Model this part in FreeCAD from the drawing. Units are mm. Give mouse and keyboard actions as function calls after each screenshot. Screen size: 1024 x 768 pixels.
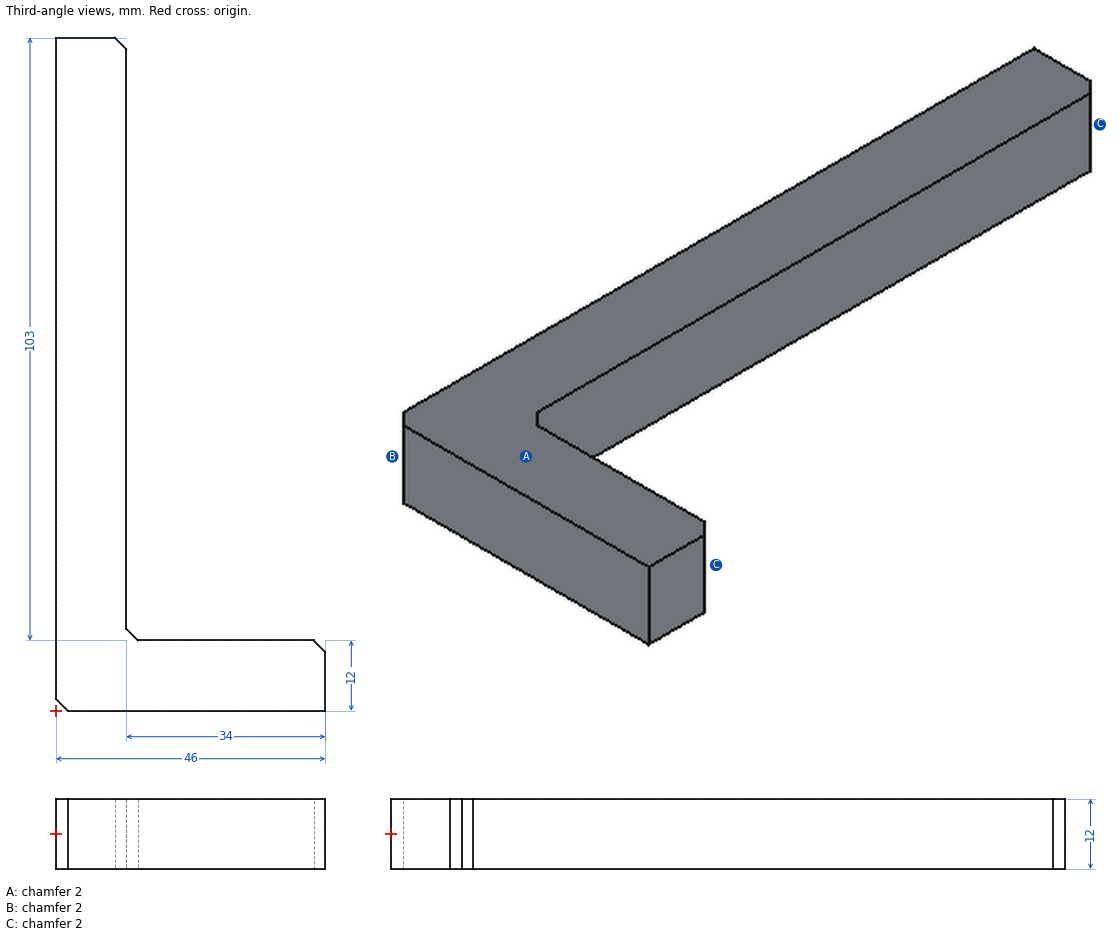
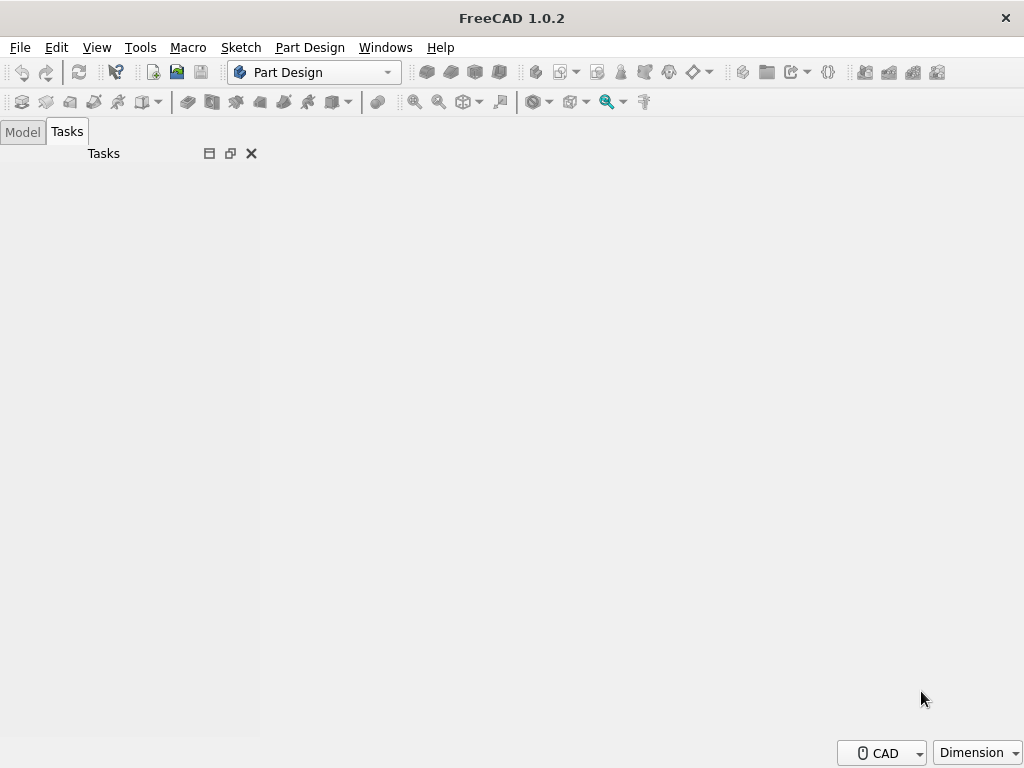
click(154, 72)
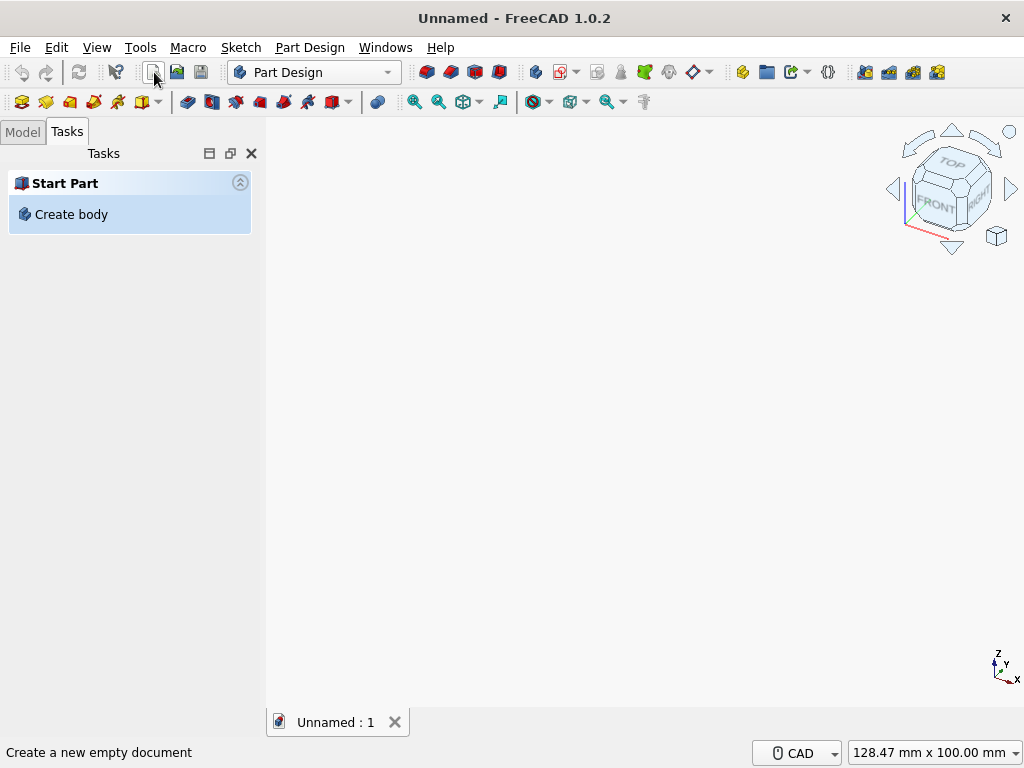
click(560, 72)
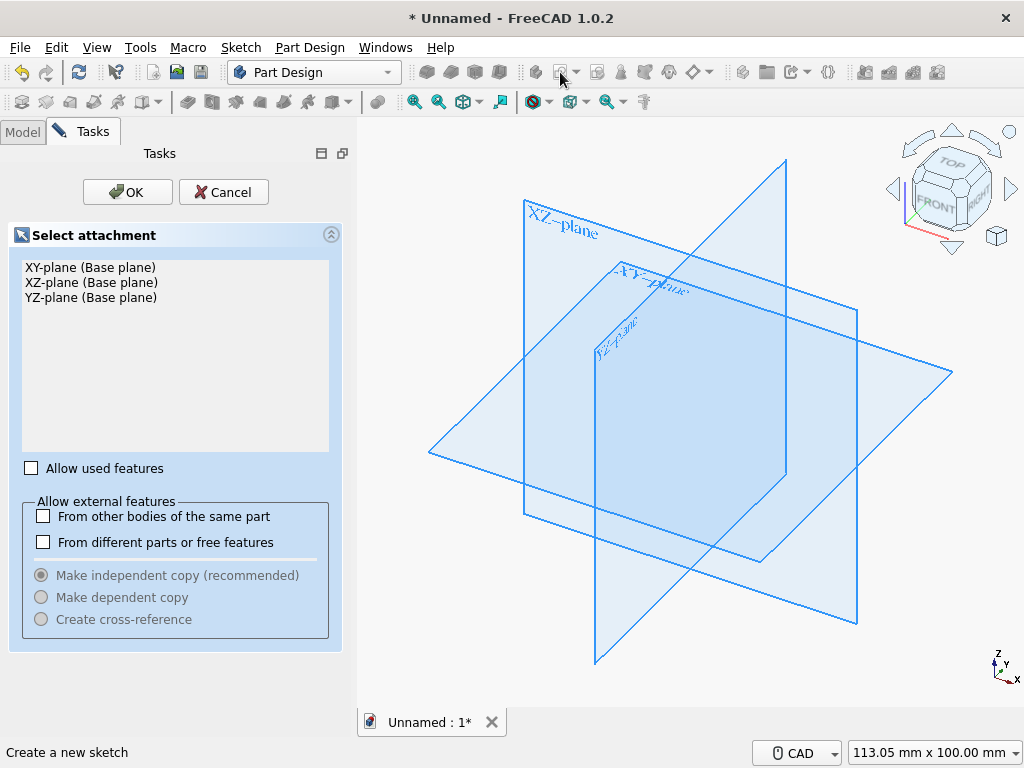
click(82, 268)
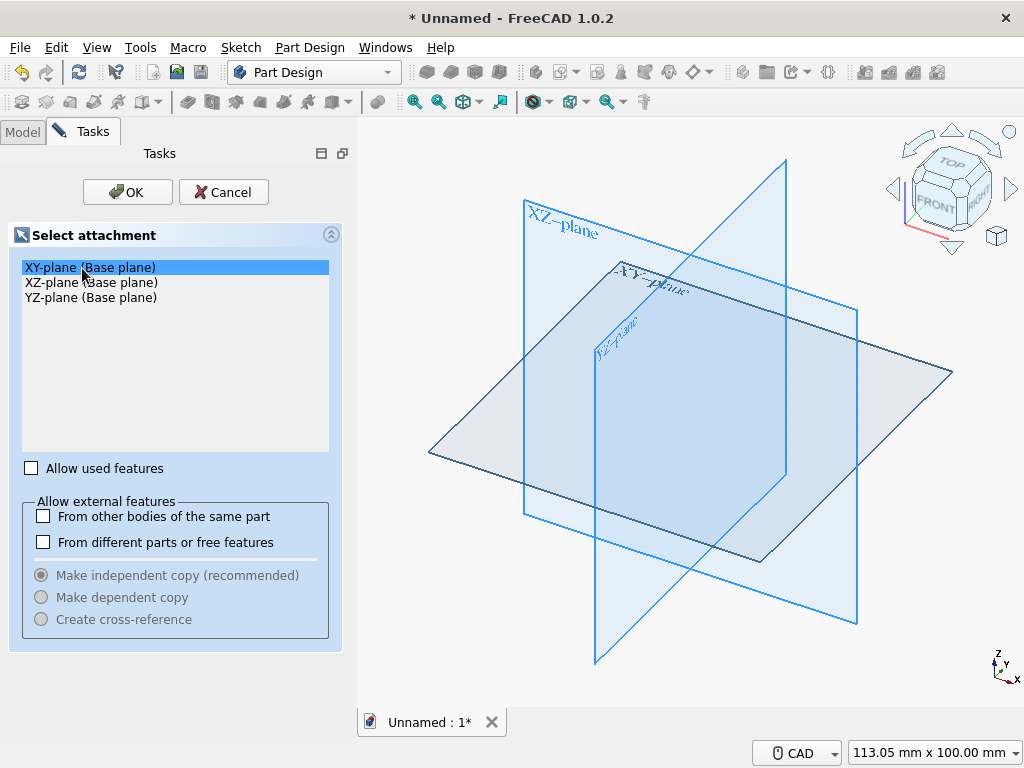
click(128, 192)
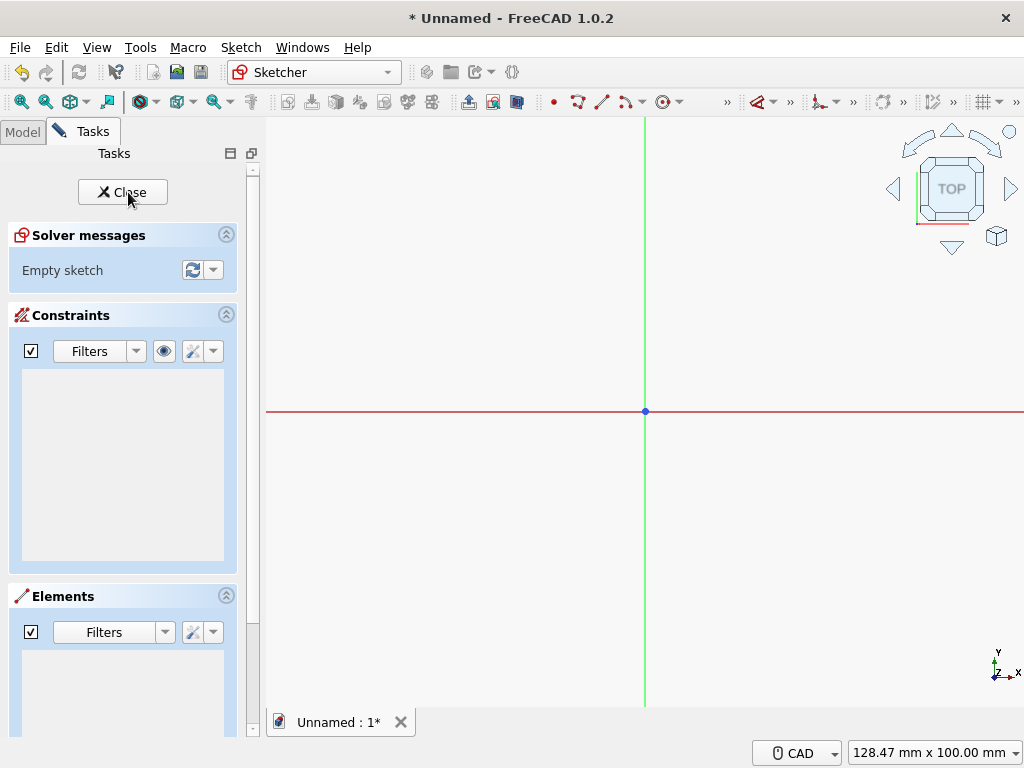
scroll(410, 679, down, 4)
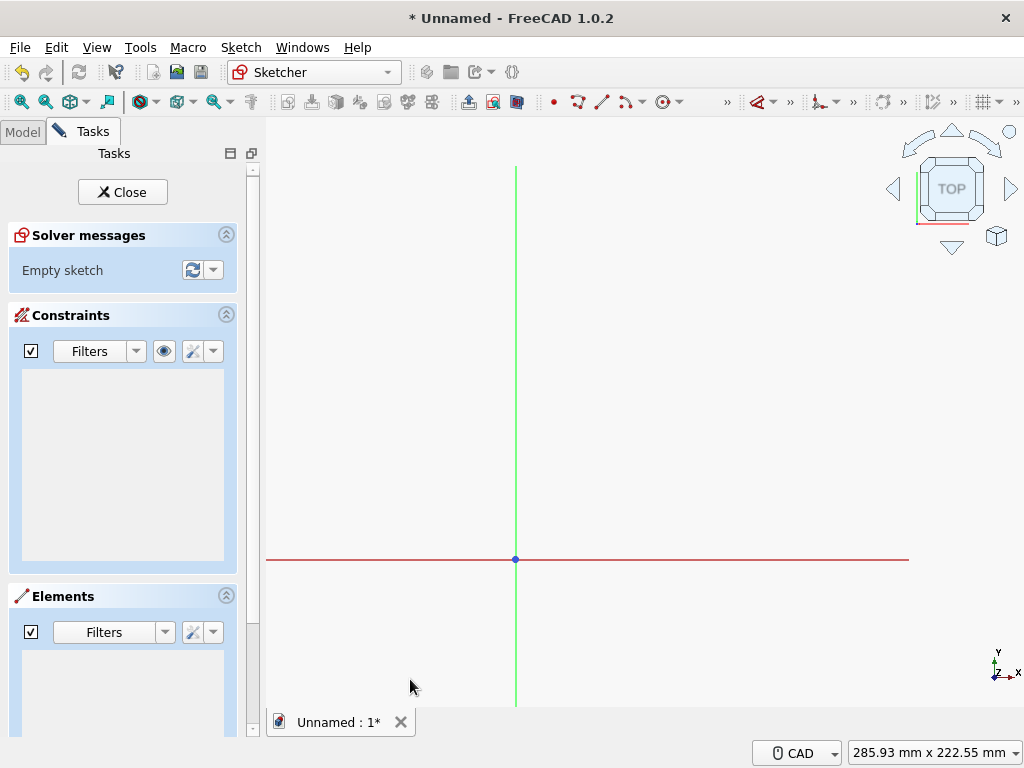
click(578, 102)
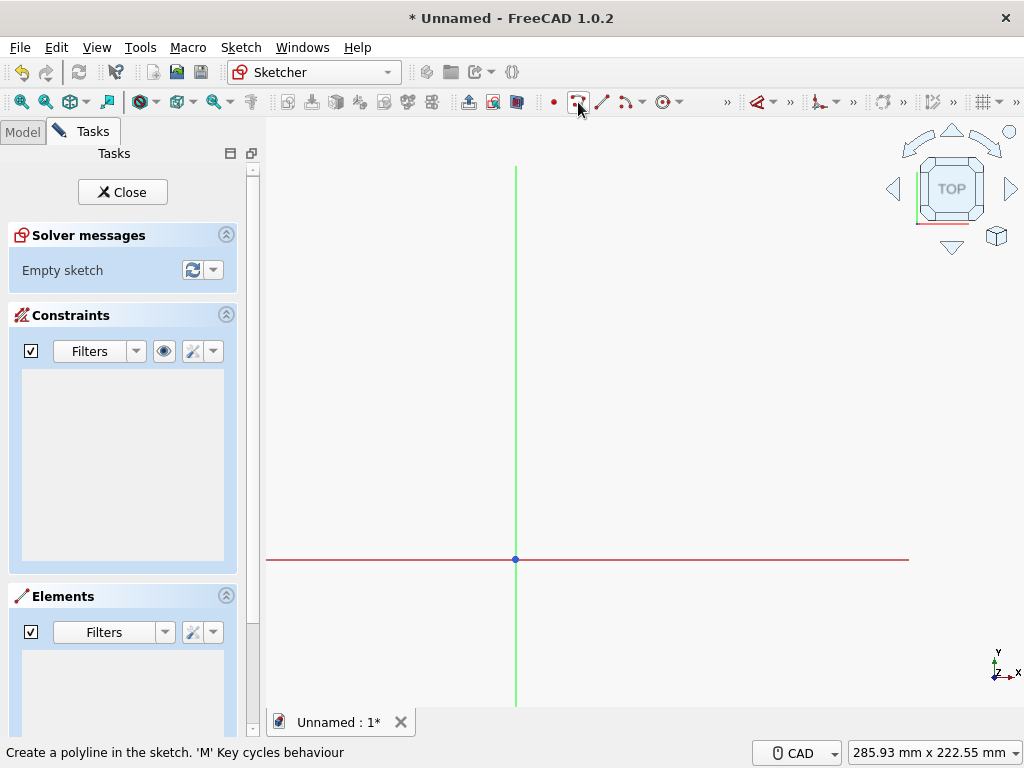
click(516, 560)
click(638, 551)
click(638, 528)
click(548, 528)
click(548, 255)
click(525, 255)
click(516, 560)
key(Escape)
key(Escape)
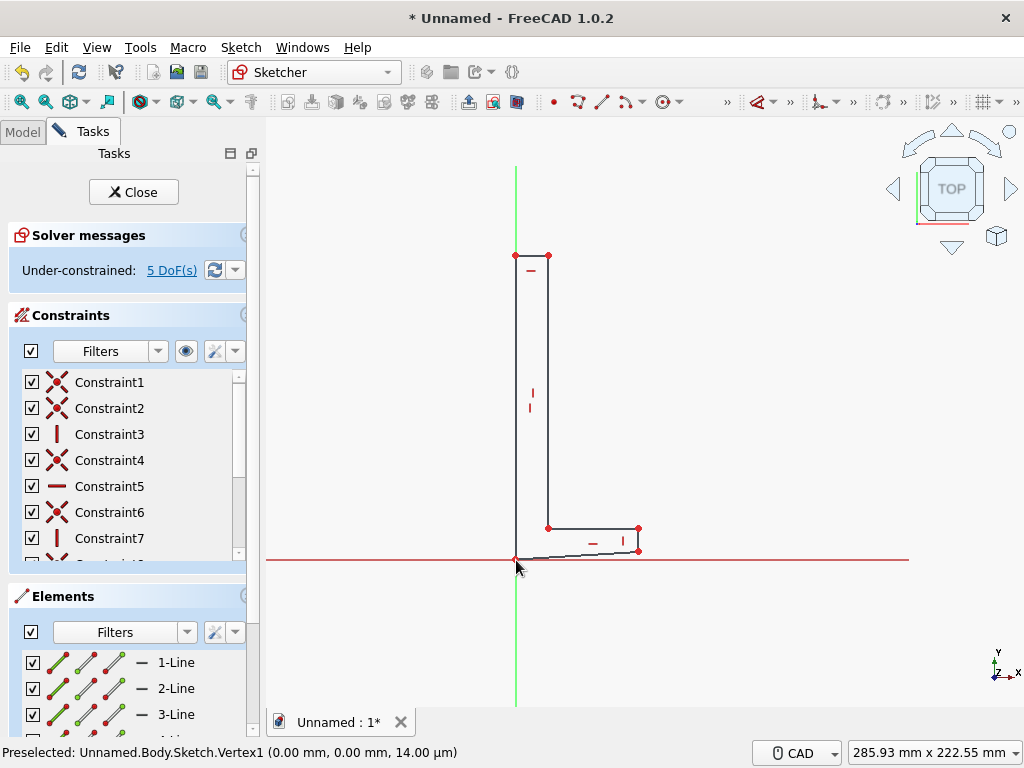
click(552, 557)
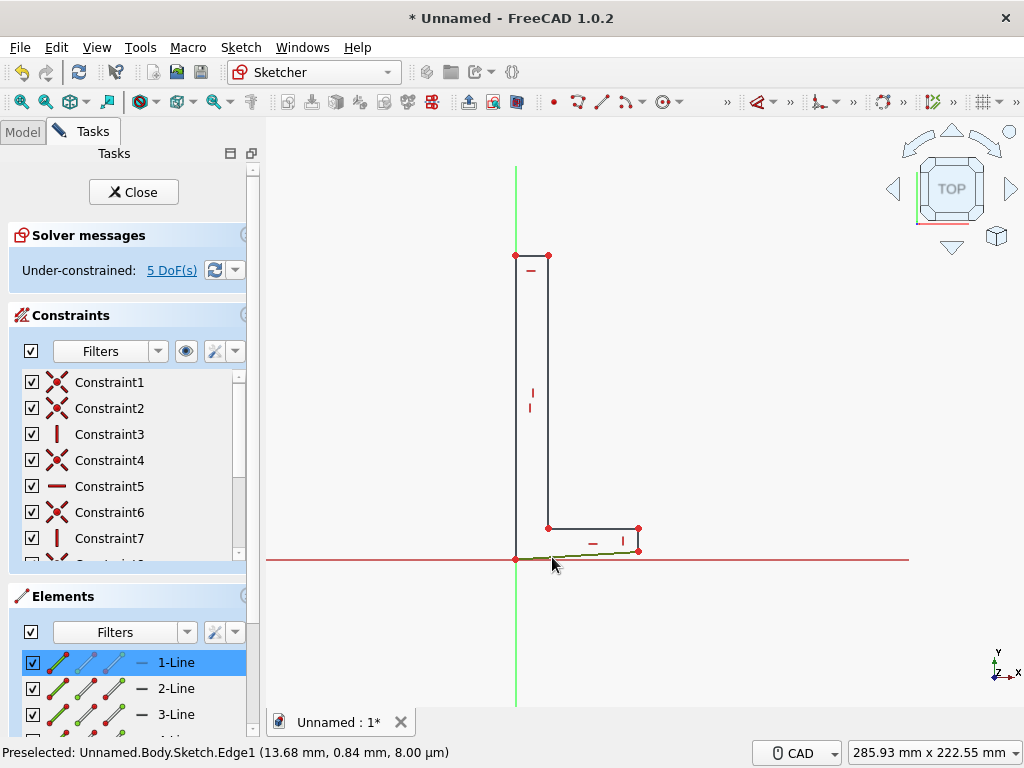
key(h)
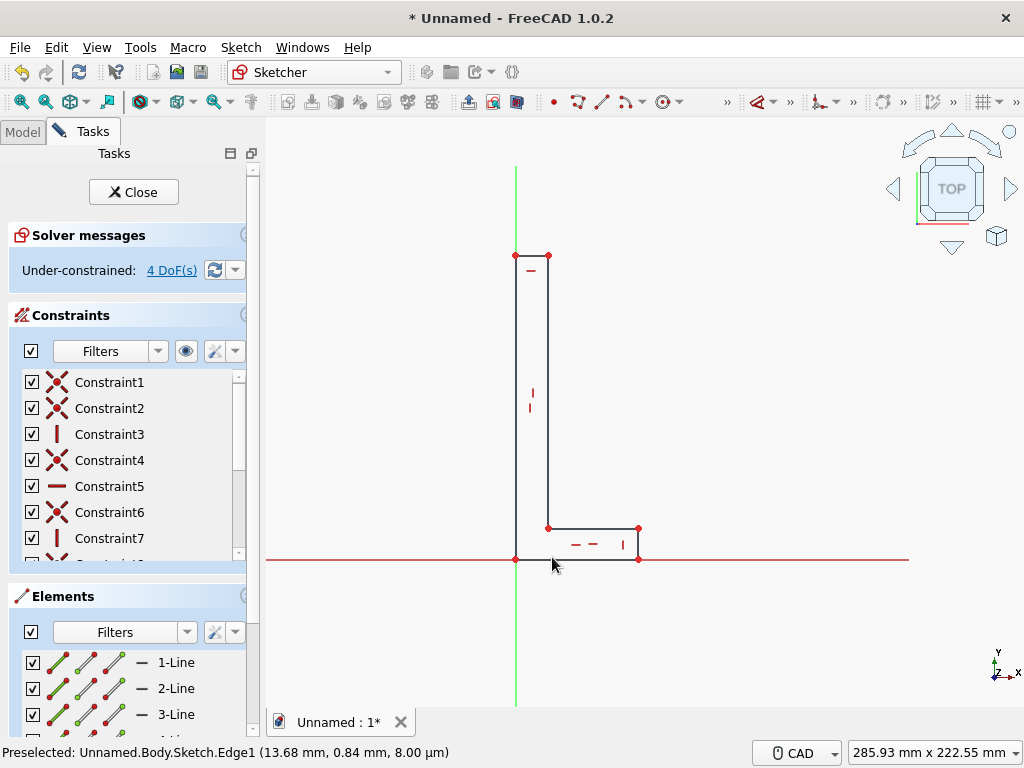
click(552, 560)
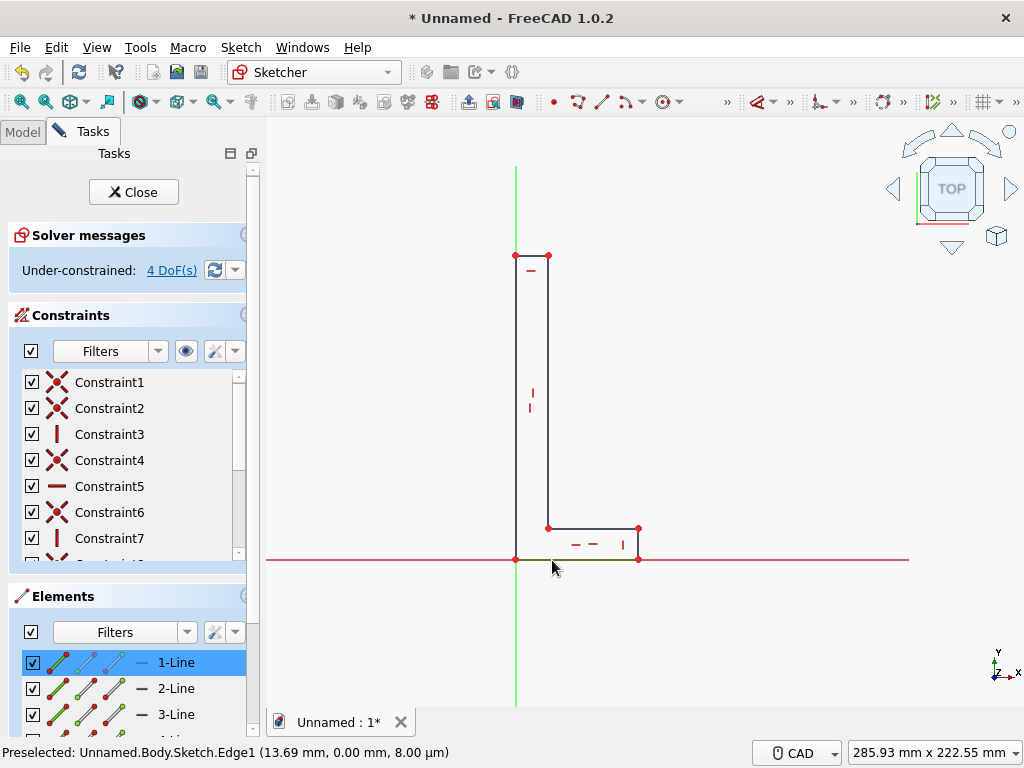
key(l)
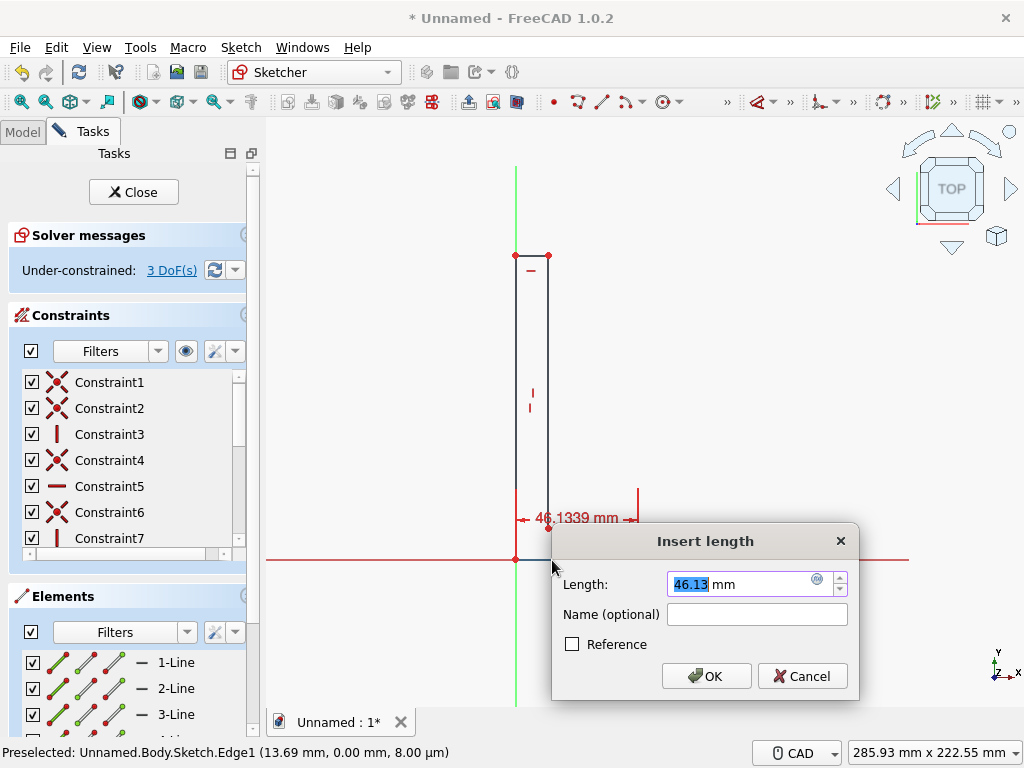
text(46)
key(Return)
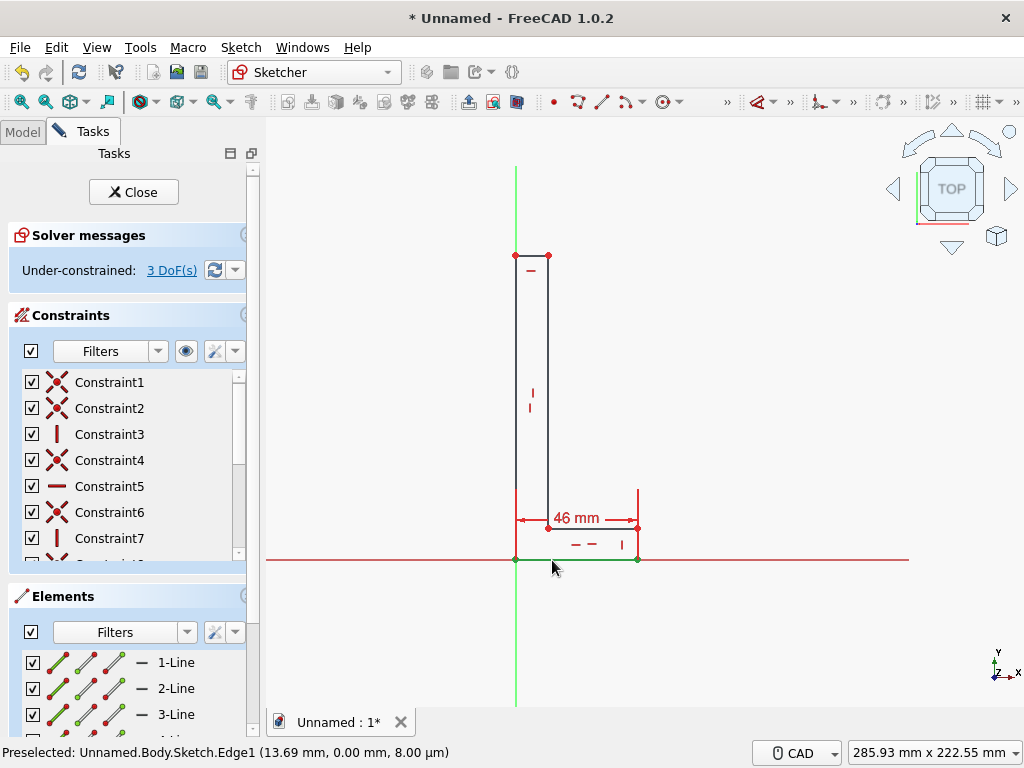
scroll(638, 550, up, 3)